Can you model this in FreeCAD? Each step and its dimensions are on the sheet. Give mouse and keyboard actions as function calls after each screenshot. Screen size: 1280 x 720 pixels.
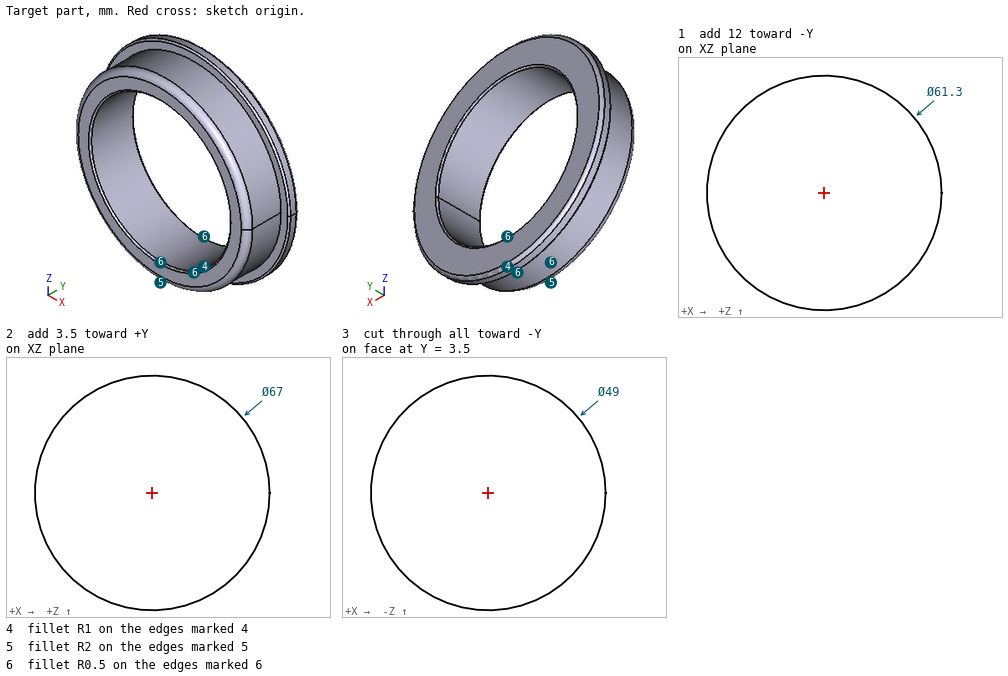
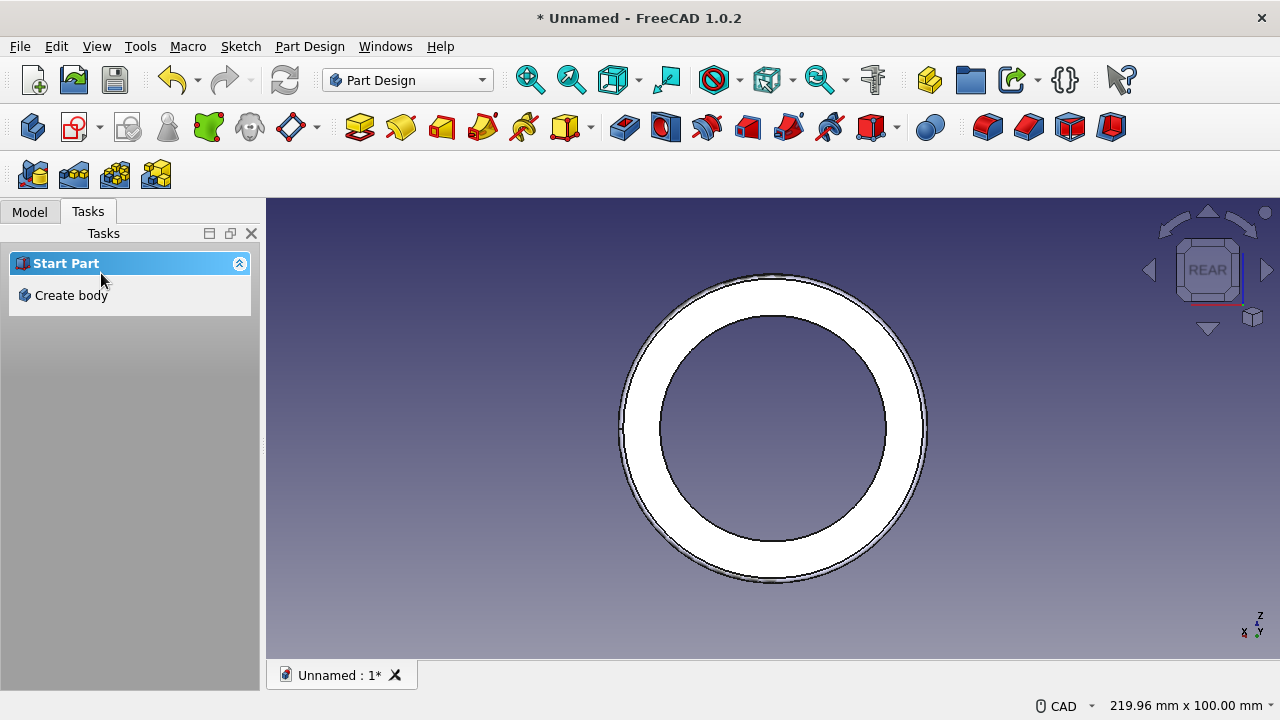
key(0)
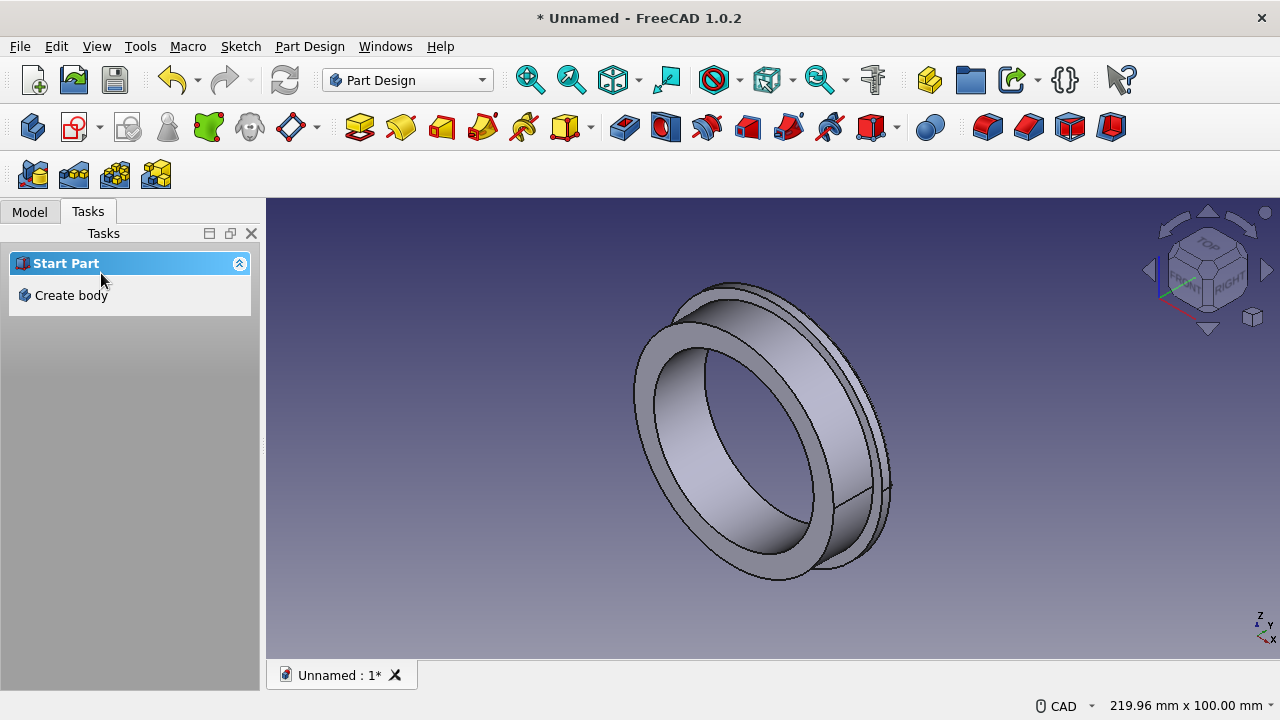
click(703, 323)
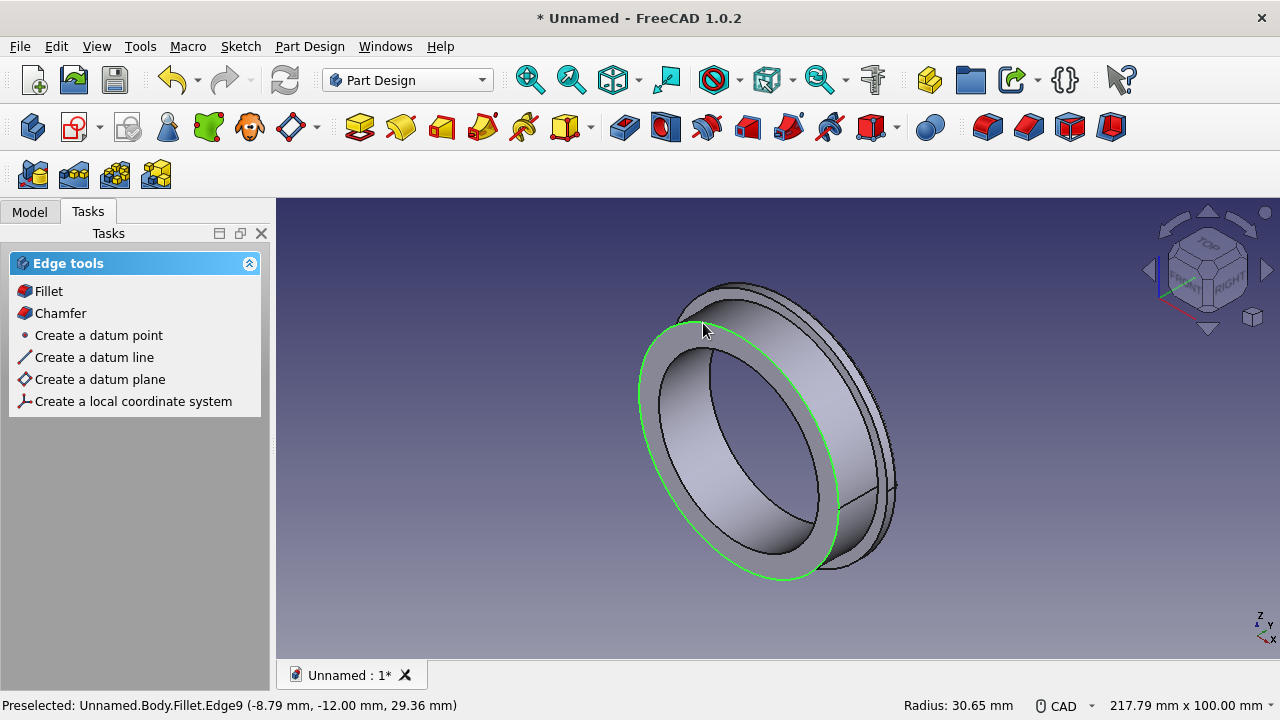
click(988, 128)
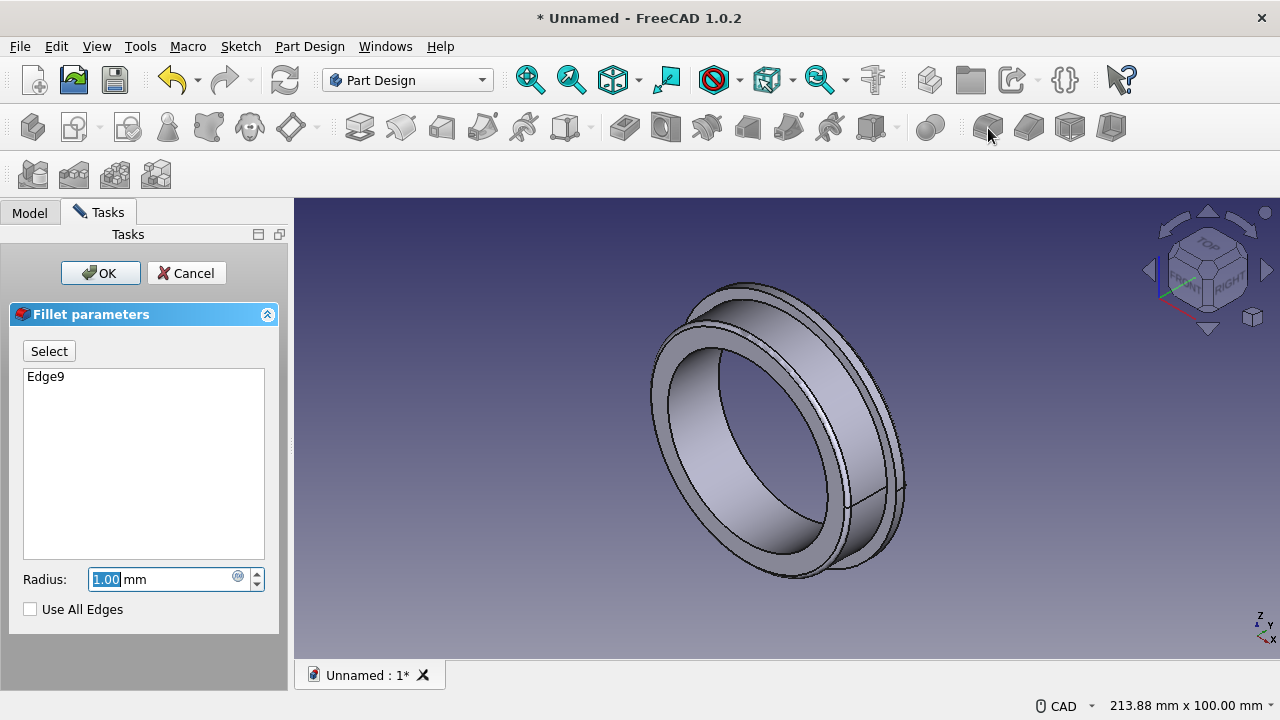
text(2)
key(Tab)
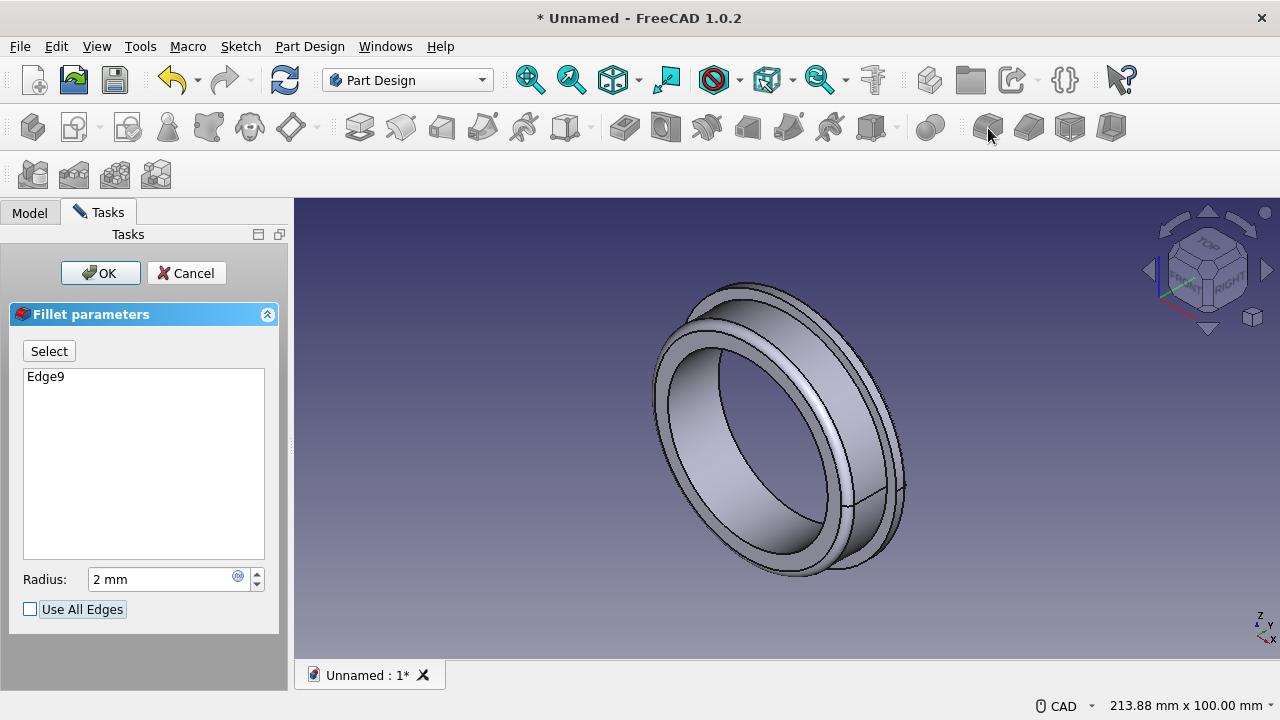
click(101, 273)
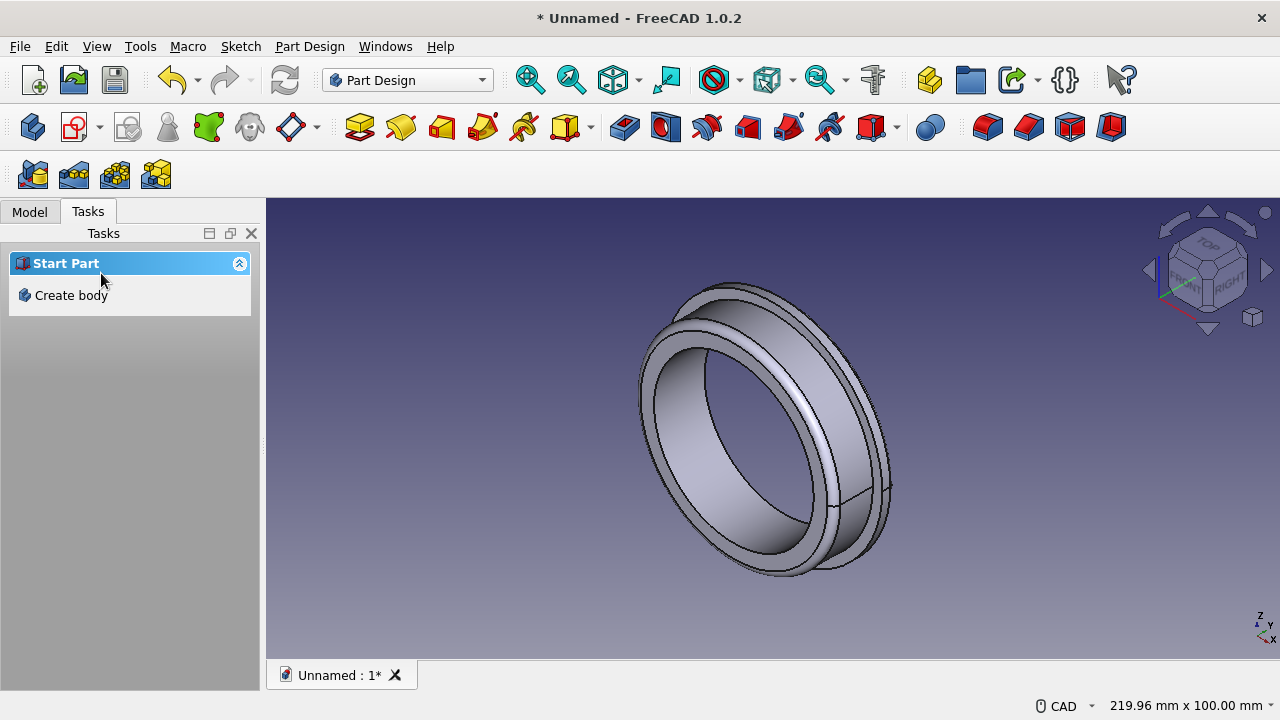
click(654, 404)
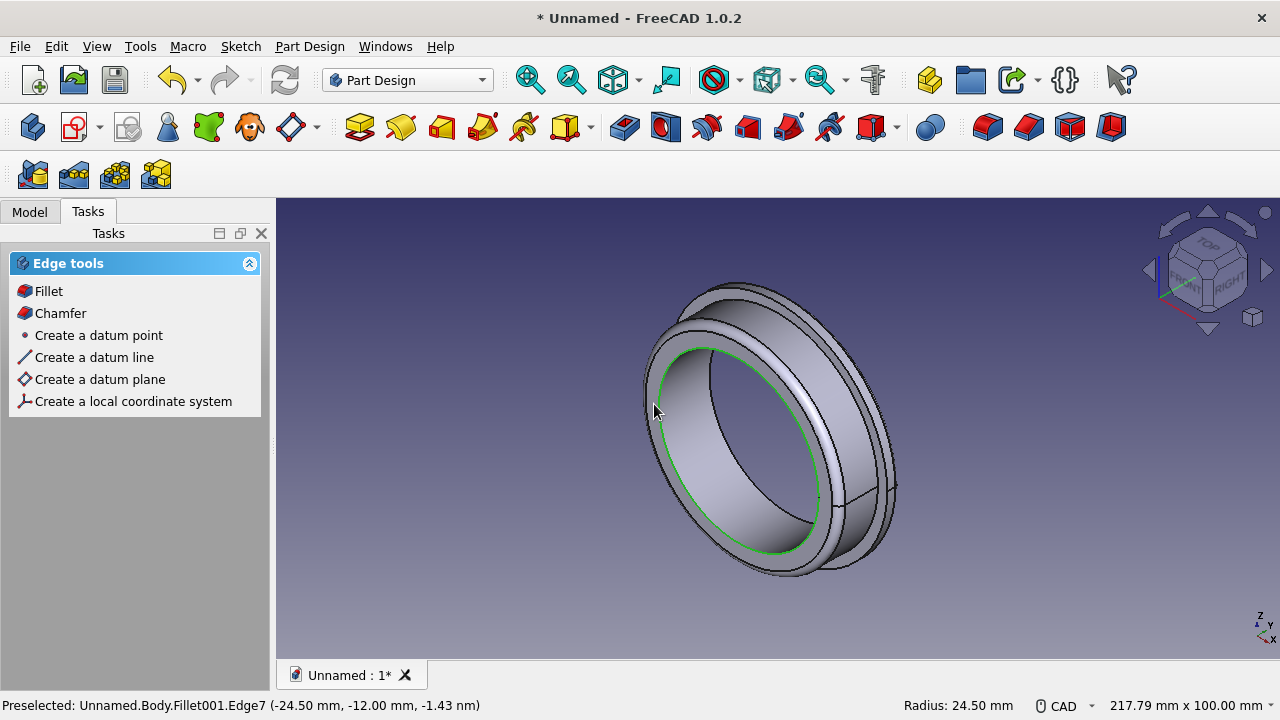
click(690, 302, ctrl)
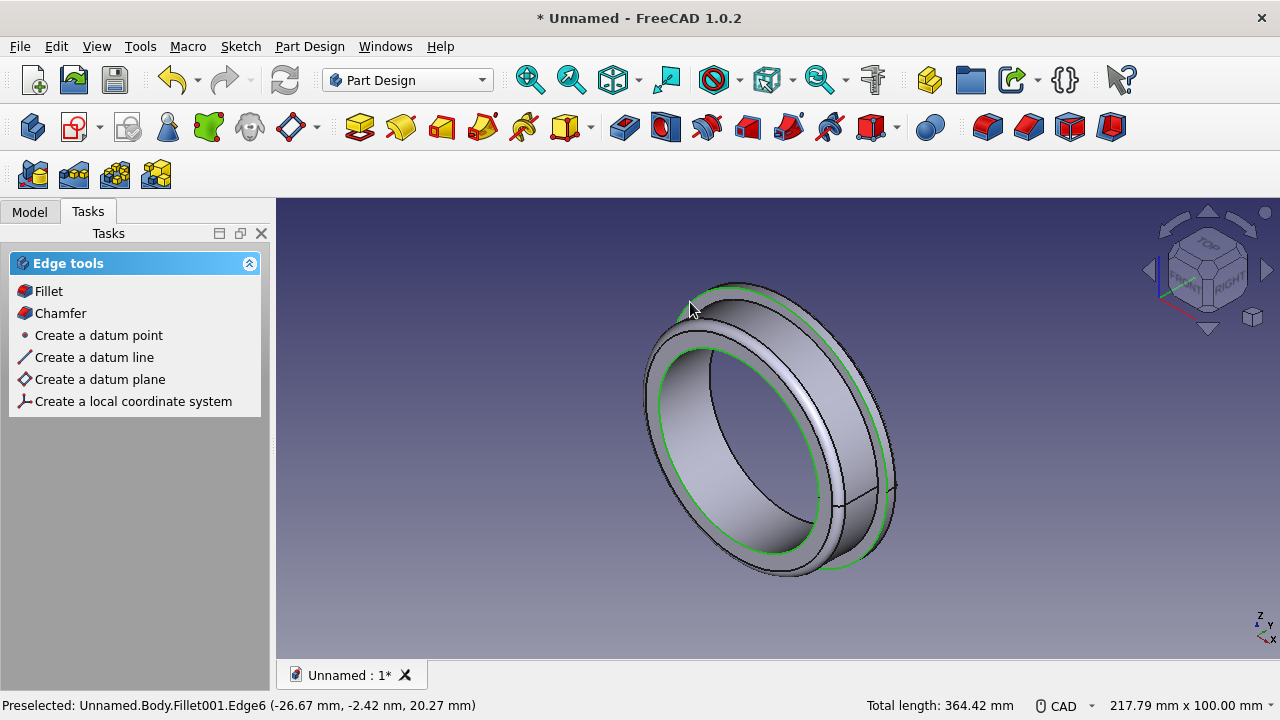
key(2)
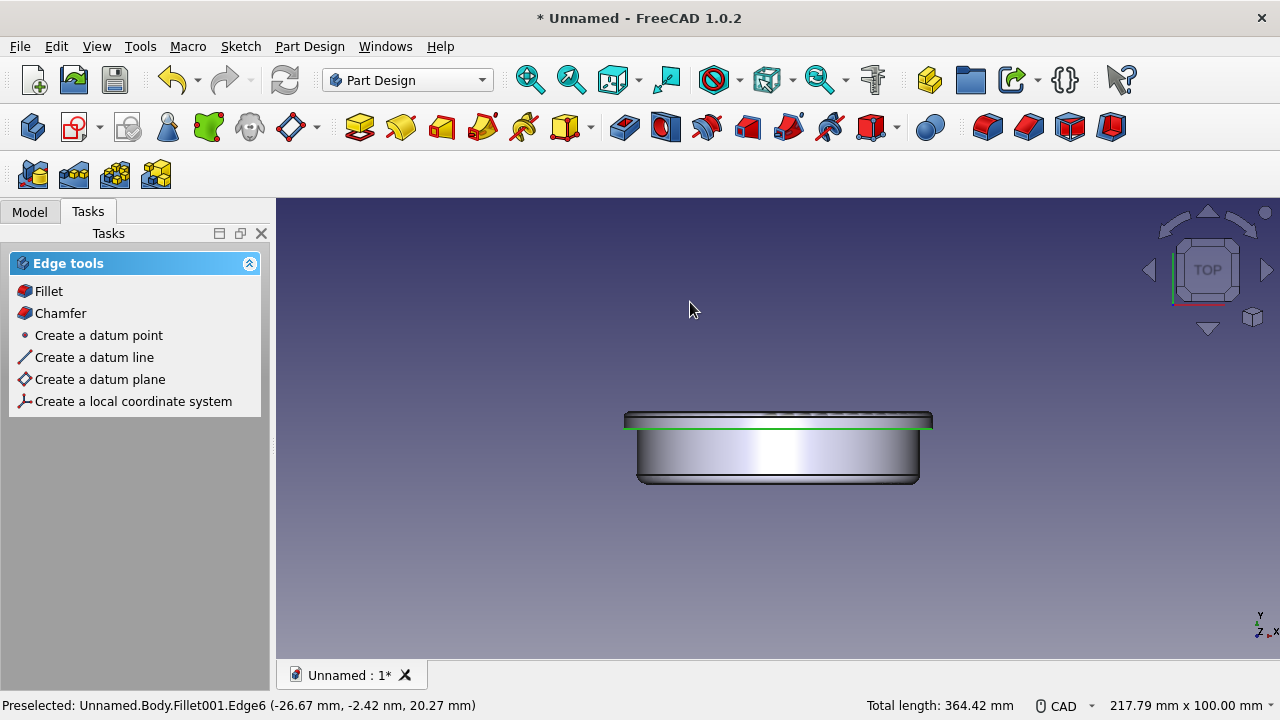
click(531, 80)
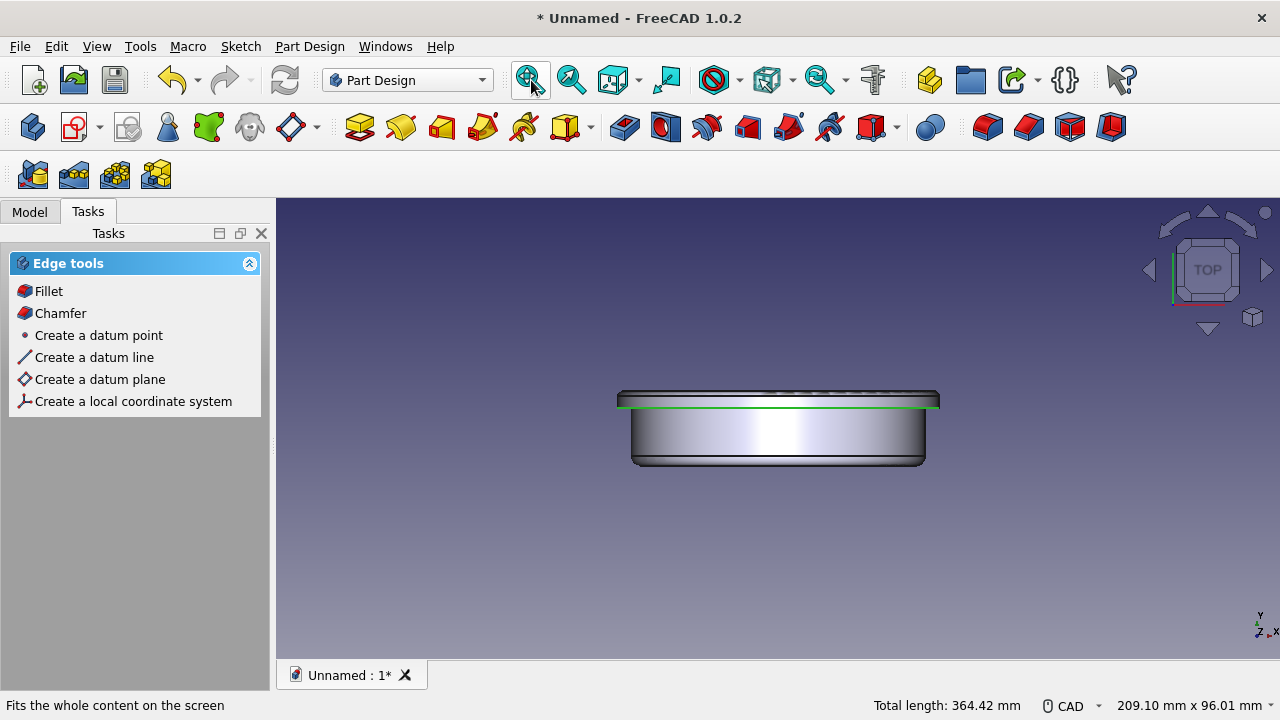
key(0)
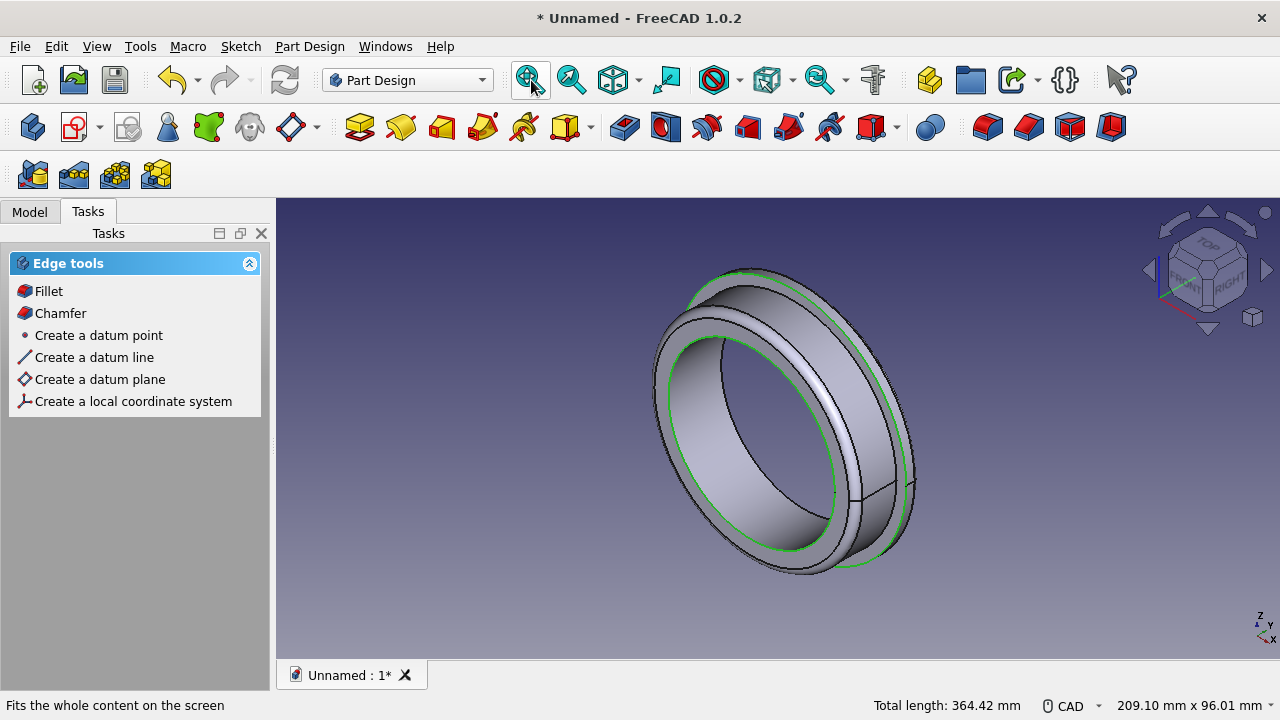
key(1)